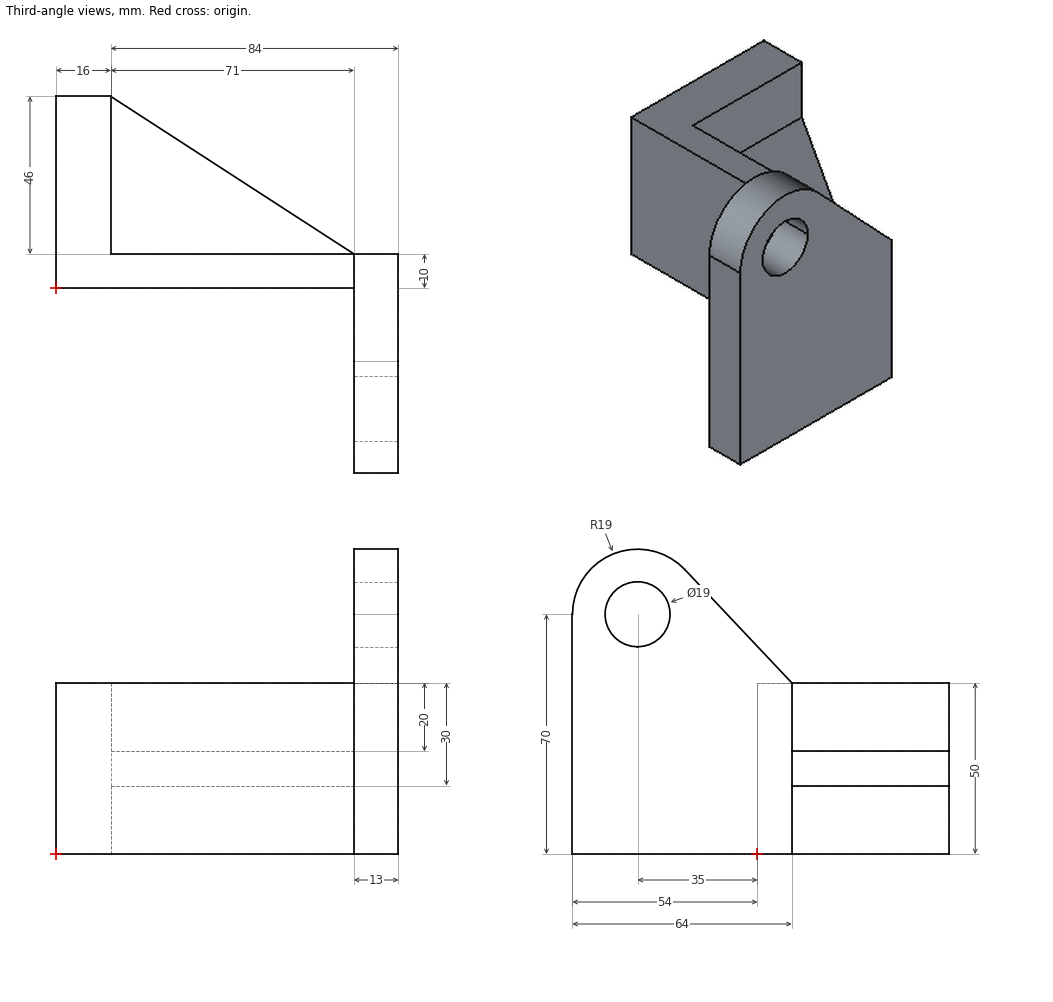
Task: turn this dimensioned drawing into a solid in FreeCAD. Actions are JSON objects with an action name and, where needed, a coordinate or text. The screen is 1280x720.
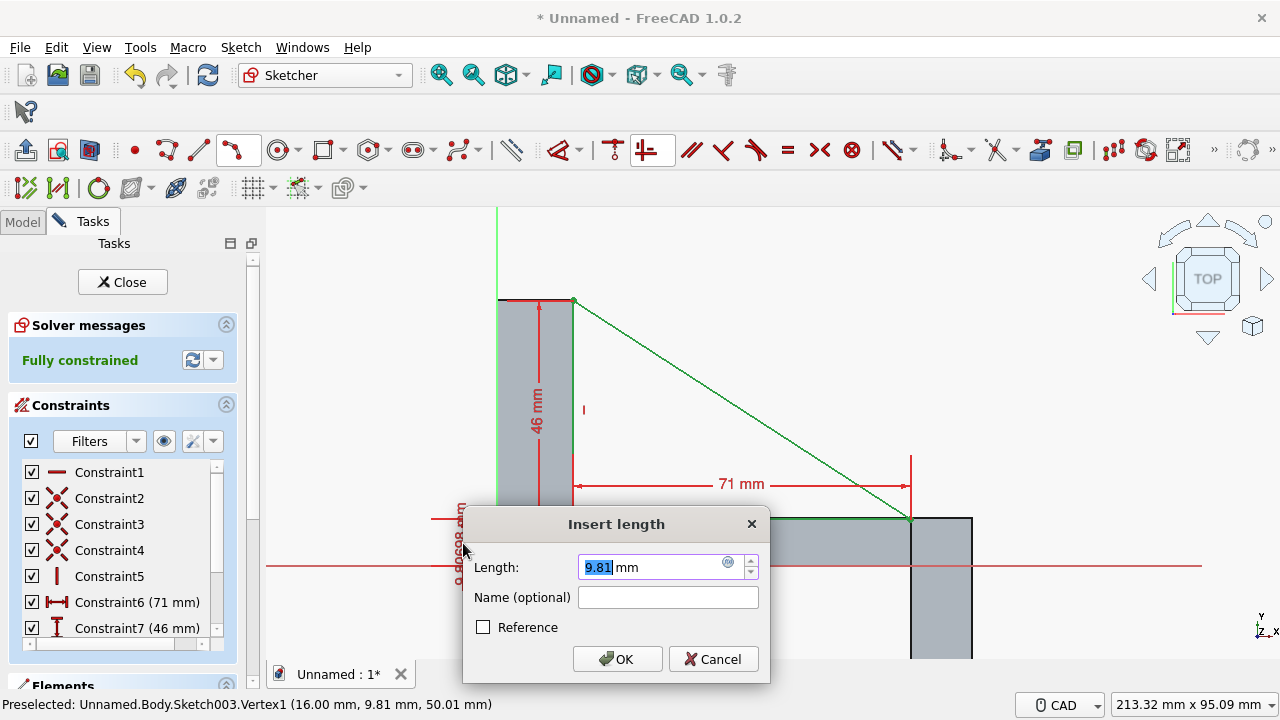
{"action": "type", "text": "10"}
{"action": "key", "text": "Return"}
{"action": "key", "text": "Escape"}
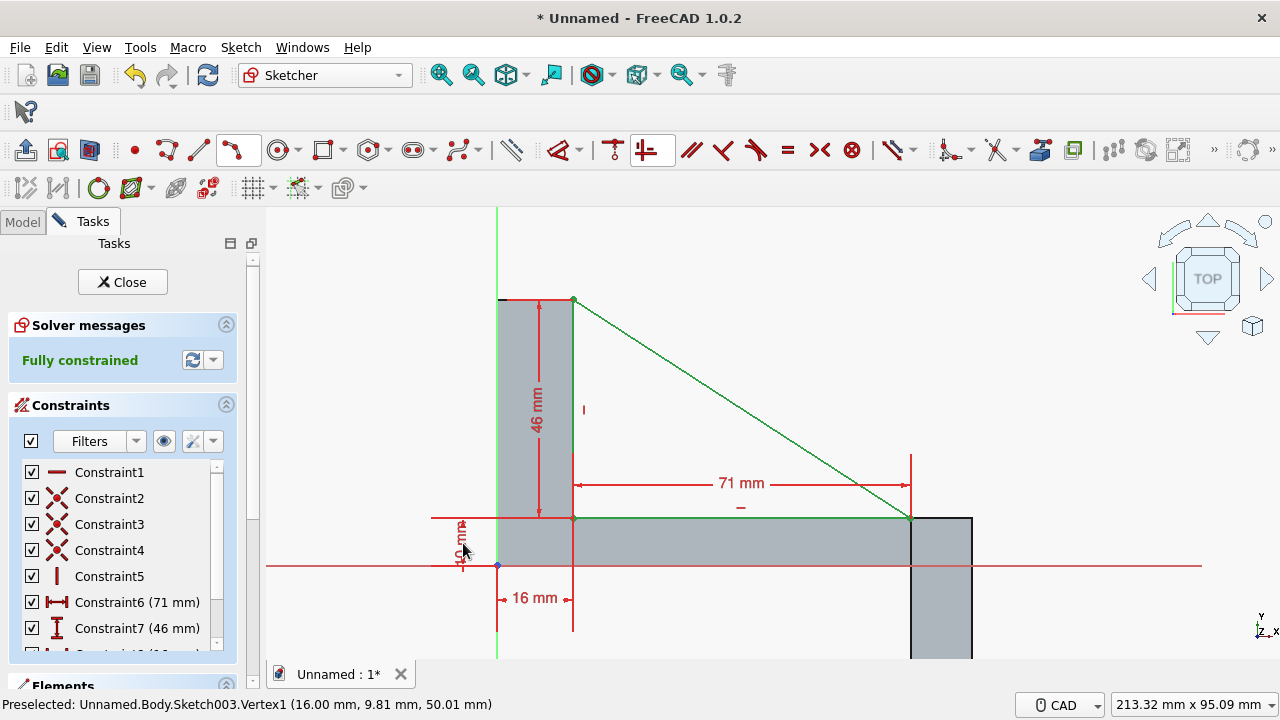
{"action": "left_click", "coordinate": [123, 282]}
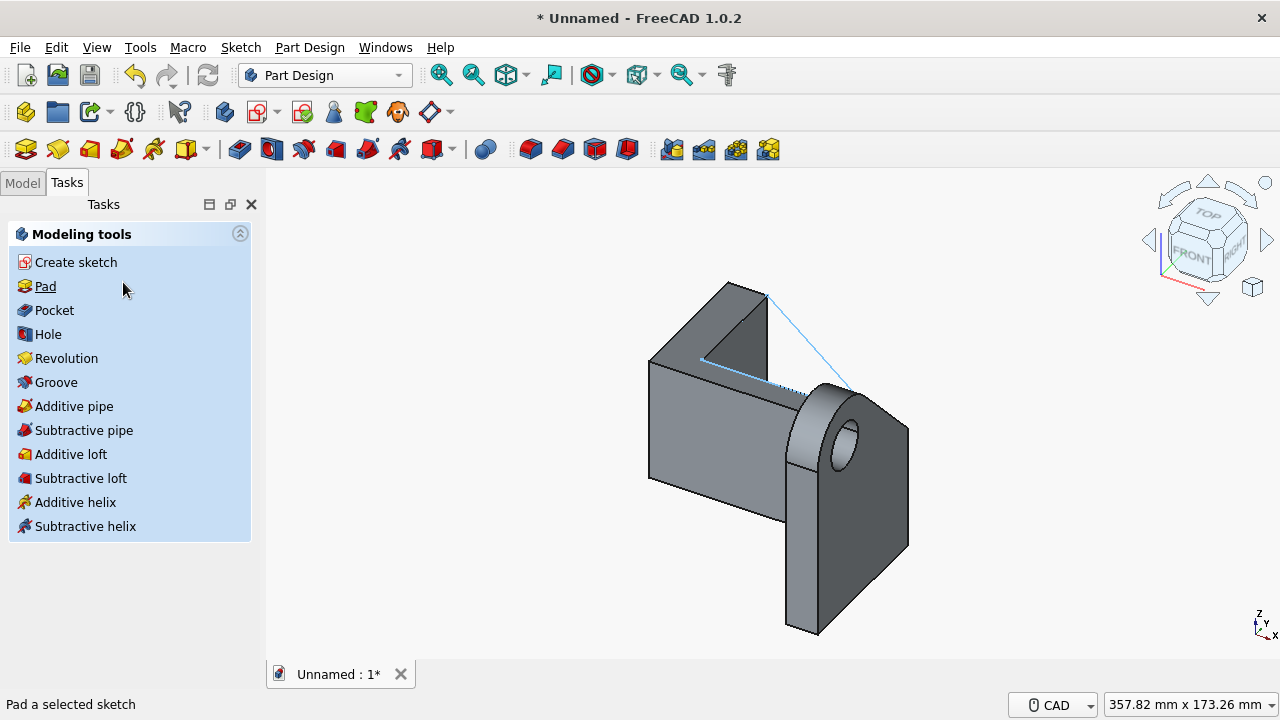
{"action": "left_click", "coordinate": [26, 150]}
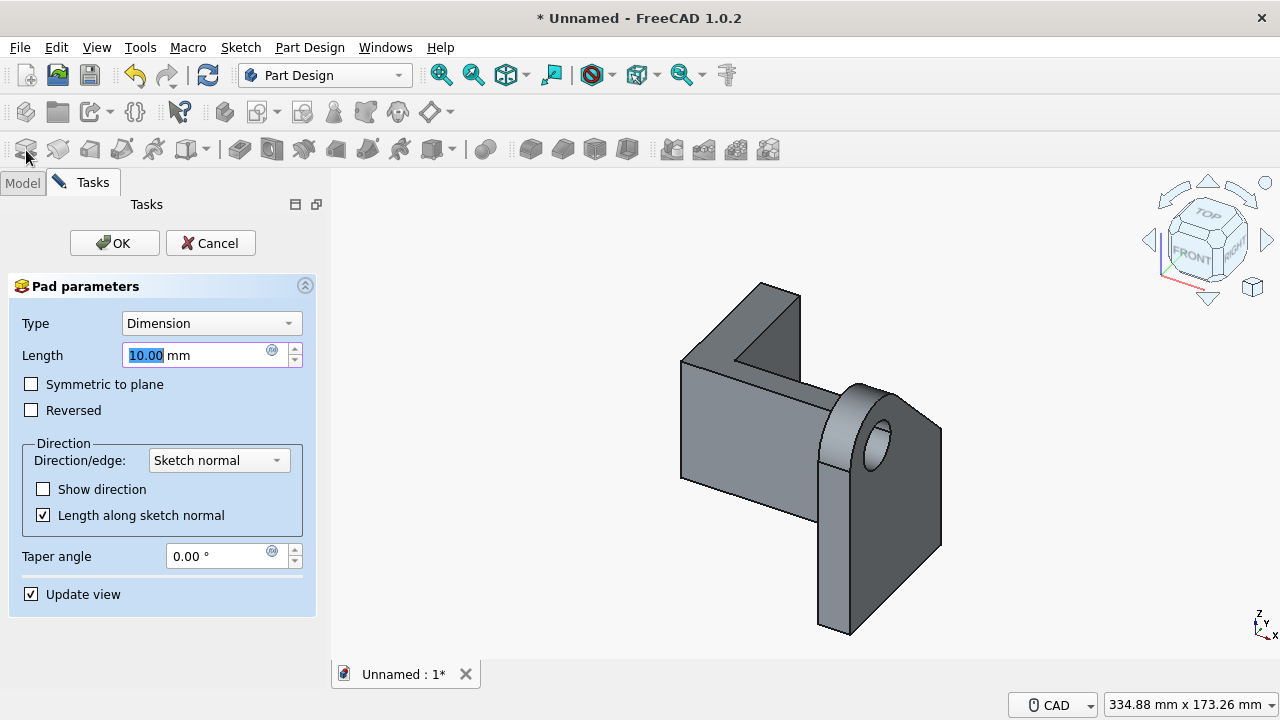
{"action": "type", "text": "30"}
{"action": "key", "text": "Tab"}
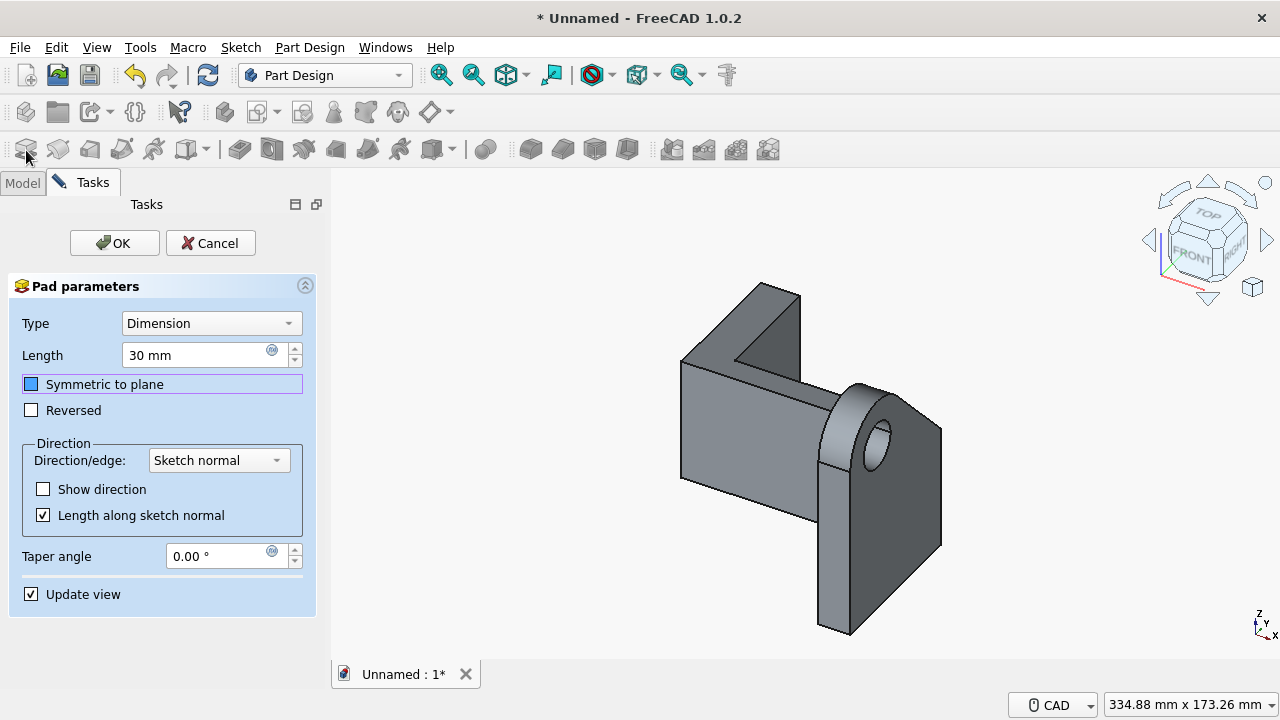
{"action": "left_click", "coordinate": [30, 410]}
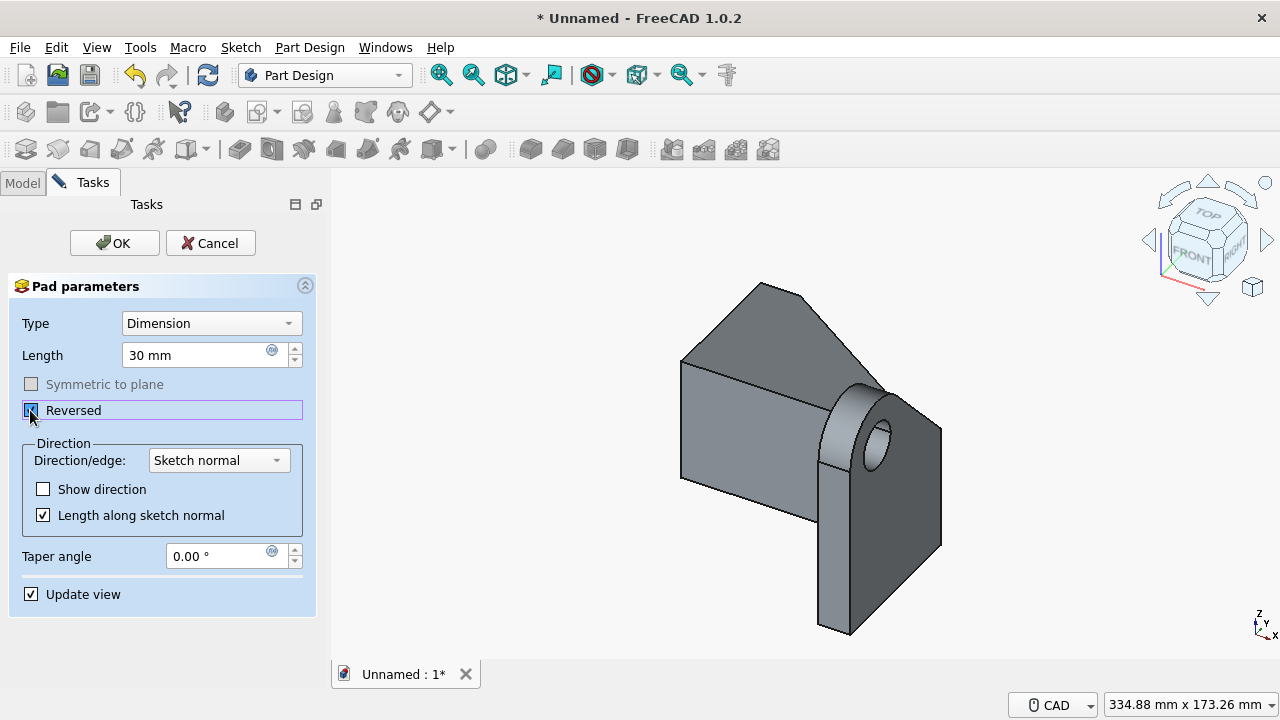
{"action": "left_click", "coordinate": [115, 243]}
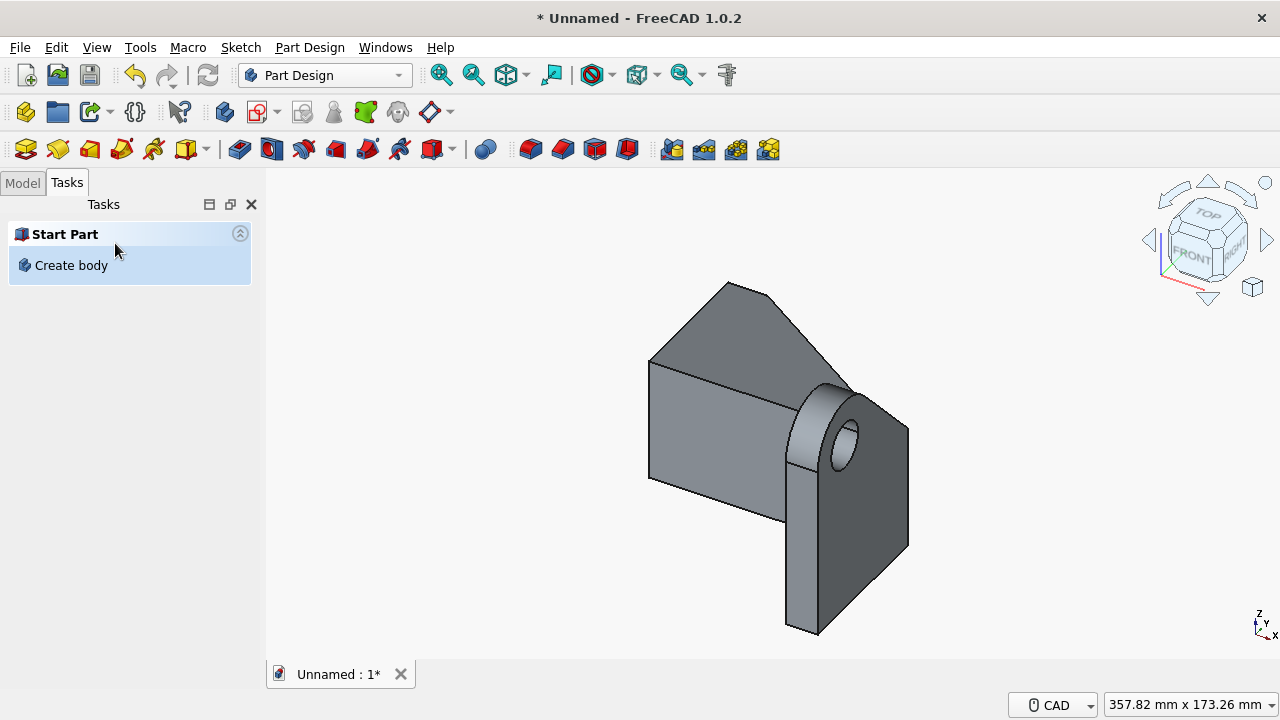
{"action": "left_click", "coordinate": [753, 358]}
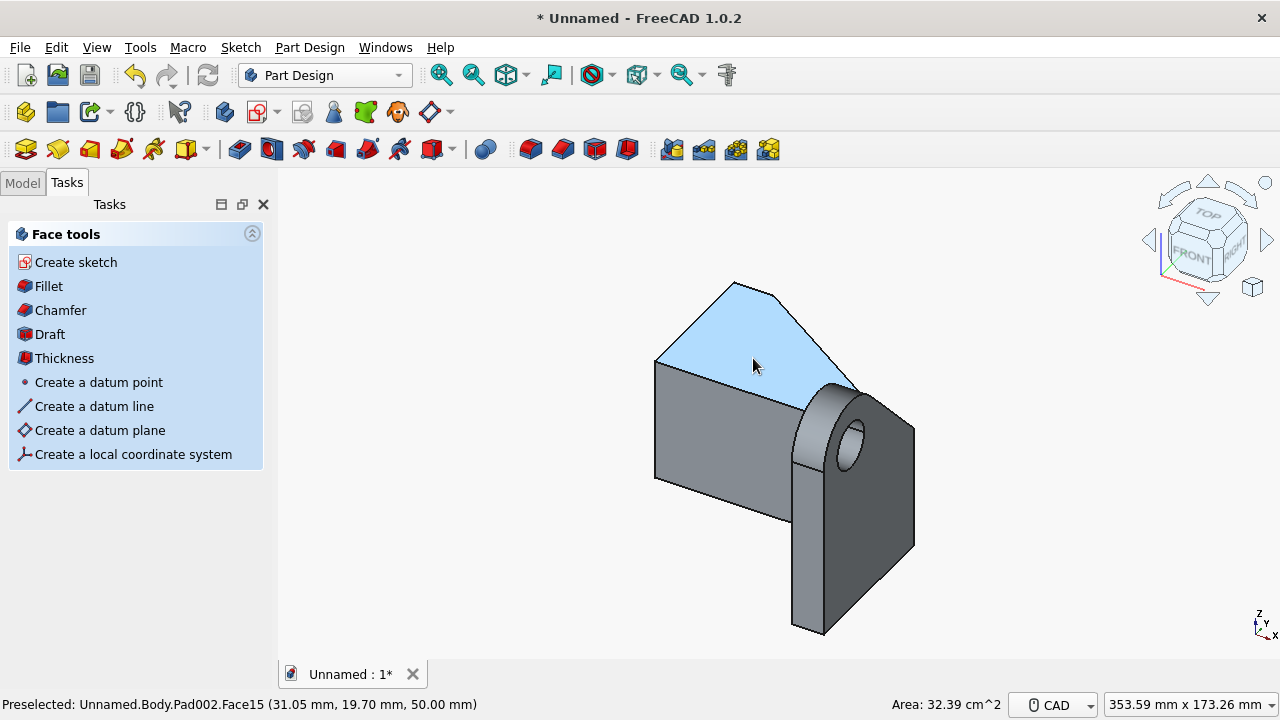
{"action": "left_click", "coordinate": [258, 112]}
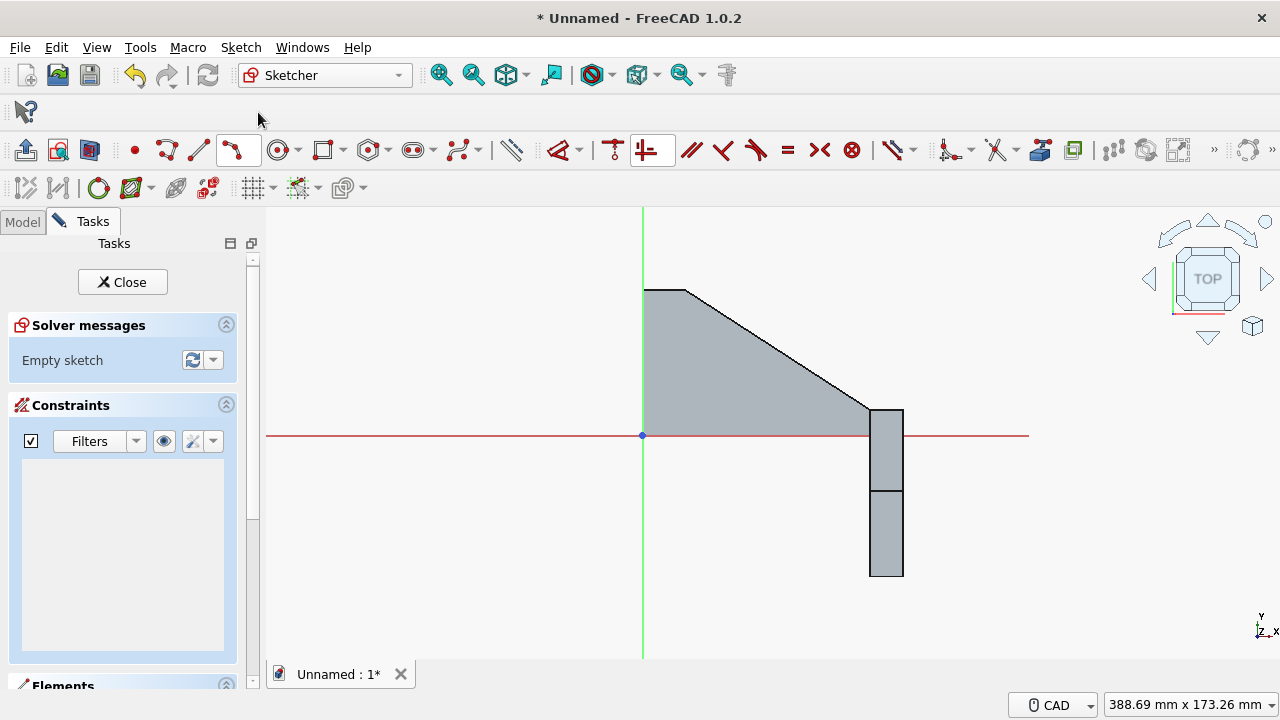
{"action": "key", "text": "q s"}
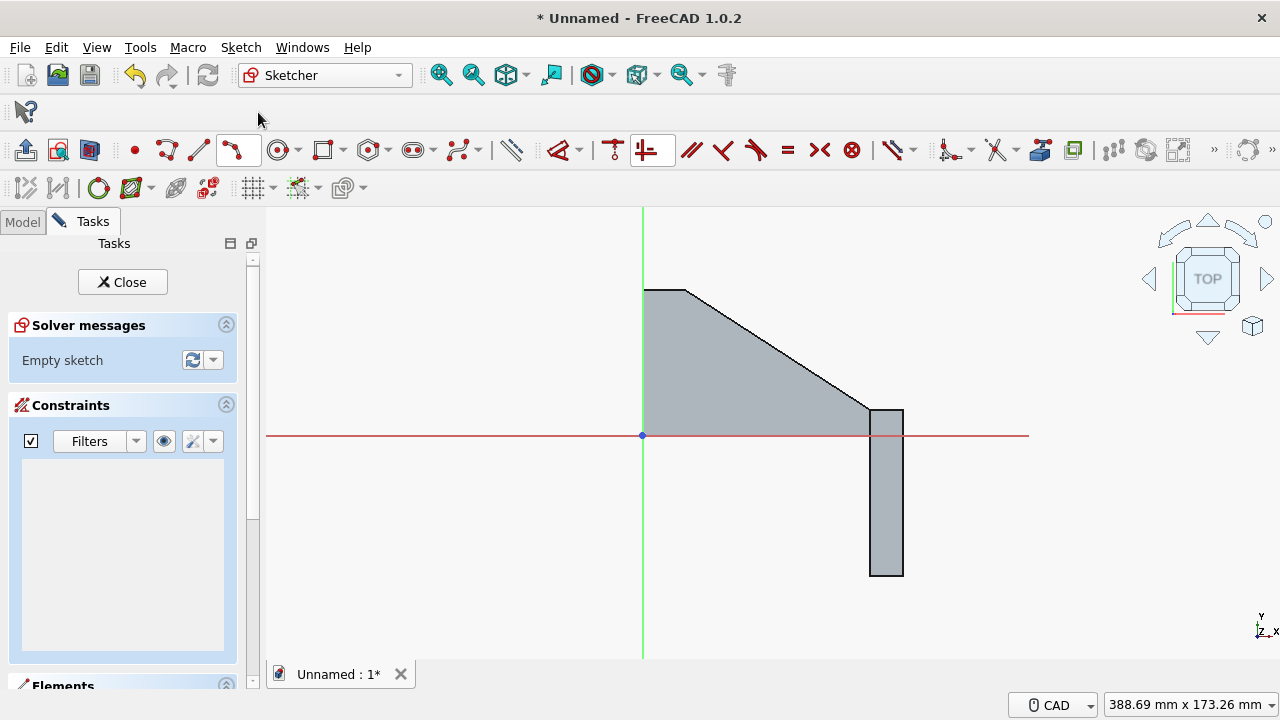
{"action": "scroll", "coordinate": [819, 277], "scroll_direction": "up", "scroll_amount": 3}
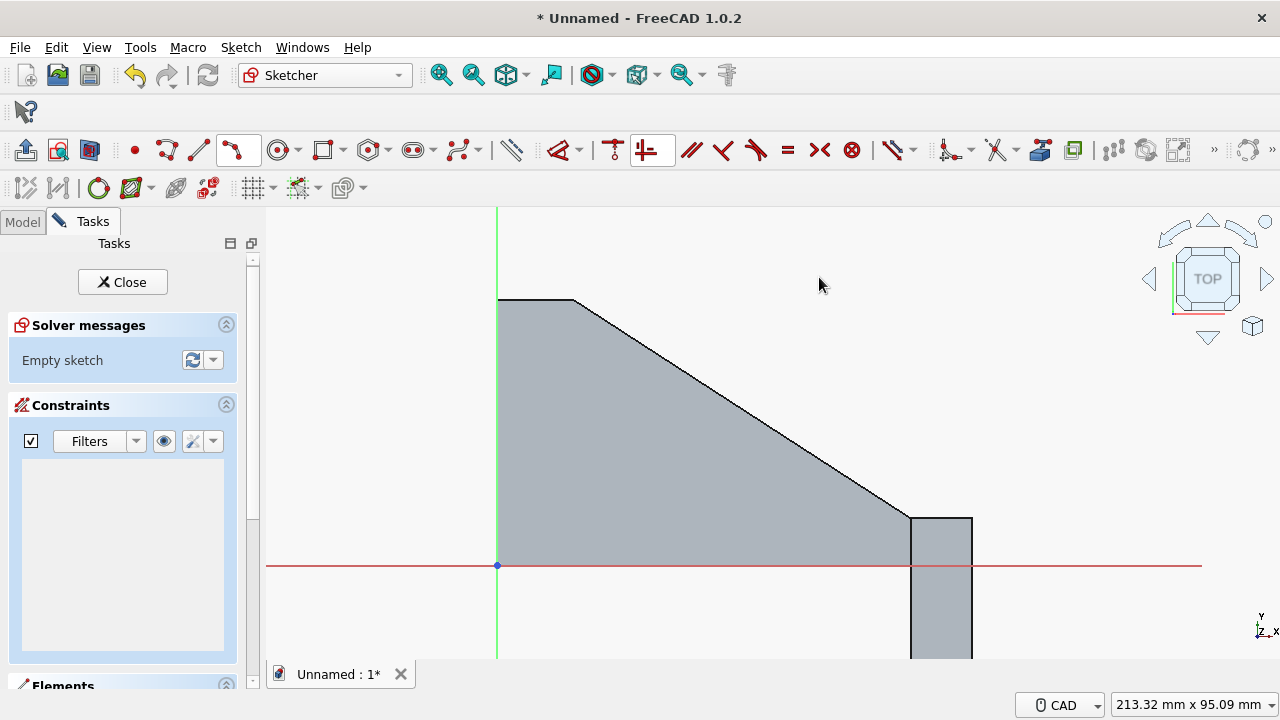
{"action": "left_click", "coordinate": [168, 150]}